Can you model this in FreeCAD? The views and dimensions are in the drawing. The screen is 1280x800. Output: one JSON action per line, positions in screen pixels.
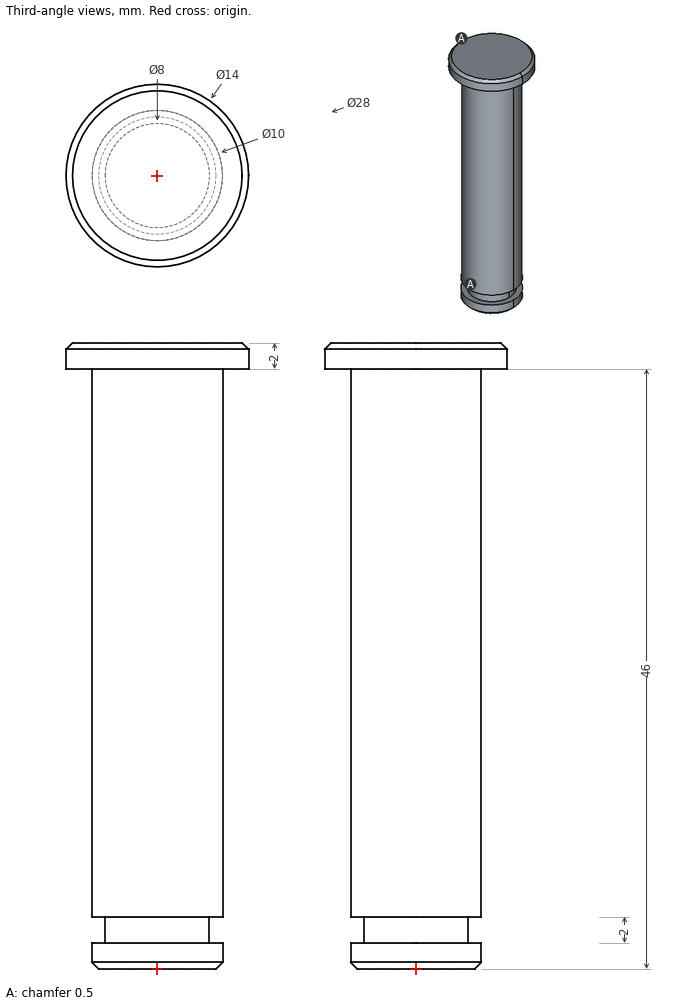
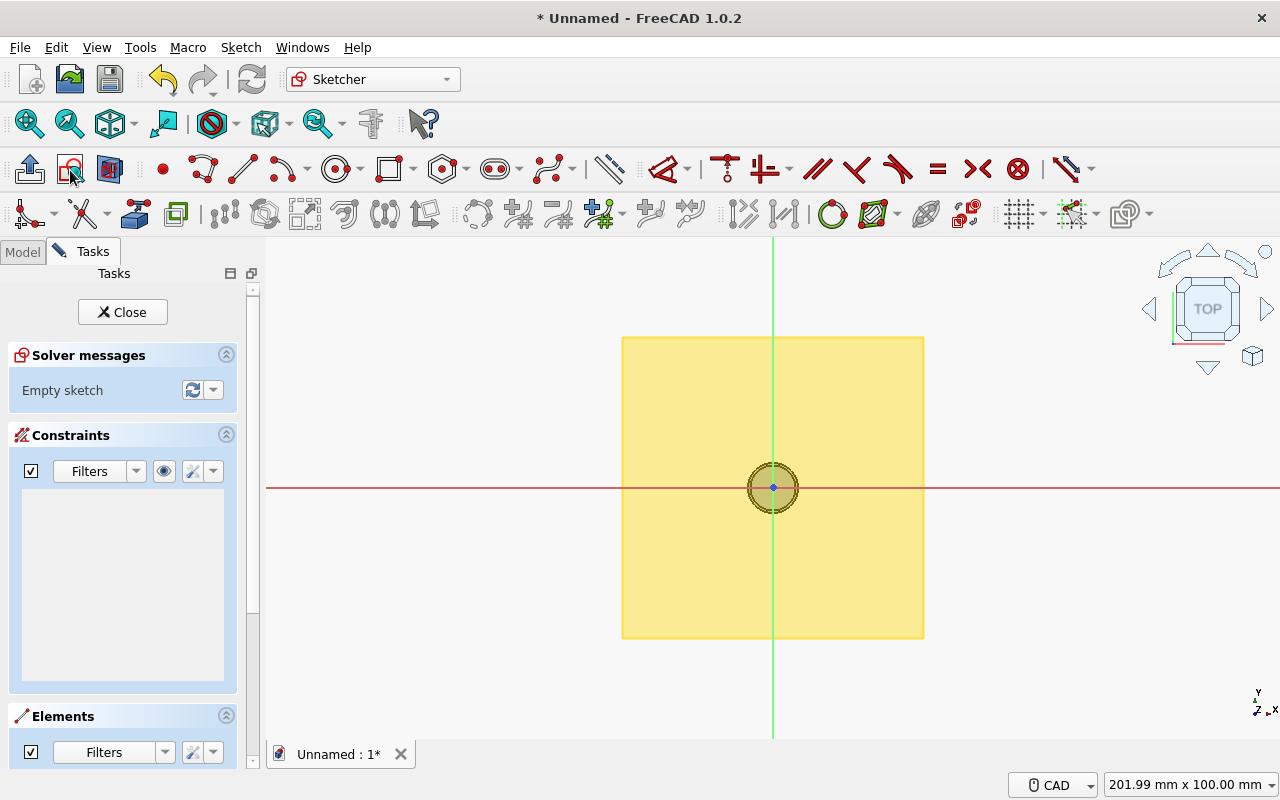
{"action": "scroll", "coordinate": [829, 488], "scroll_direction": "up", "scroll_amount": 4}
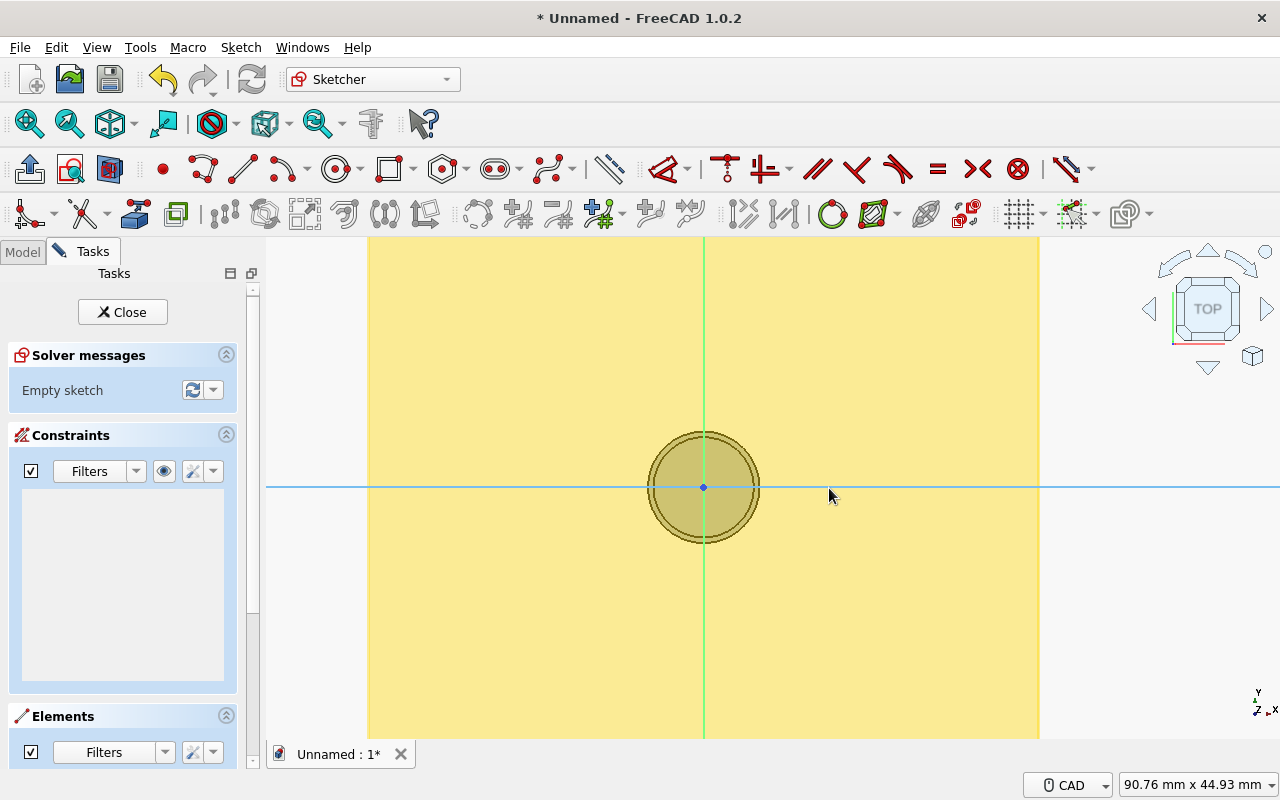
{"action": "left_click", "coordinate": [336, 170]}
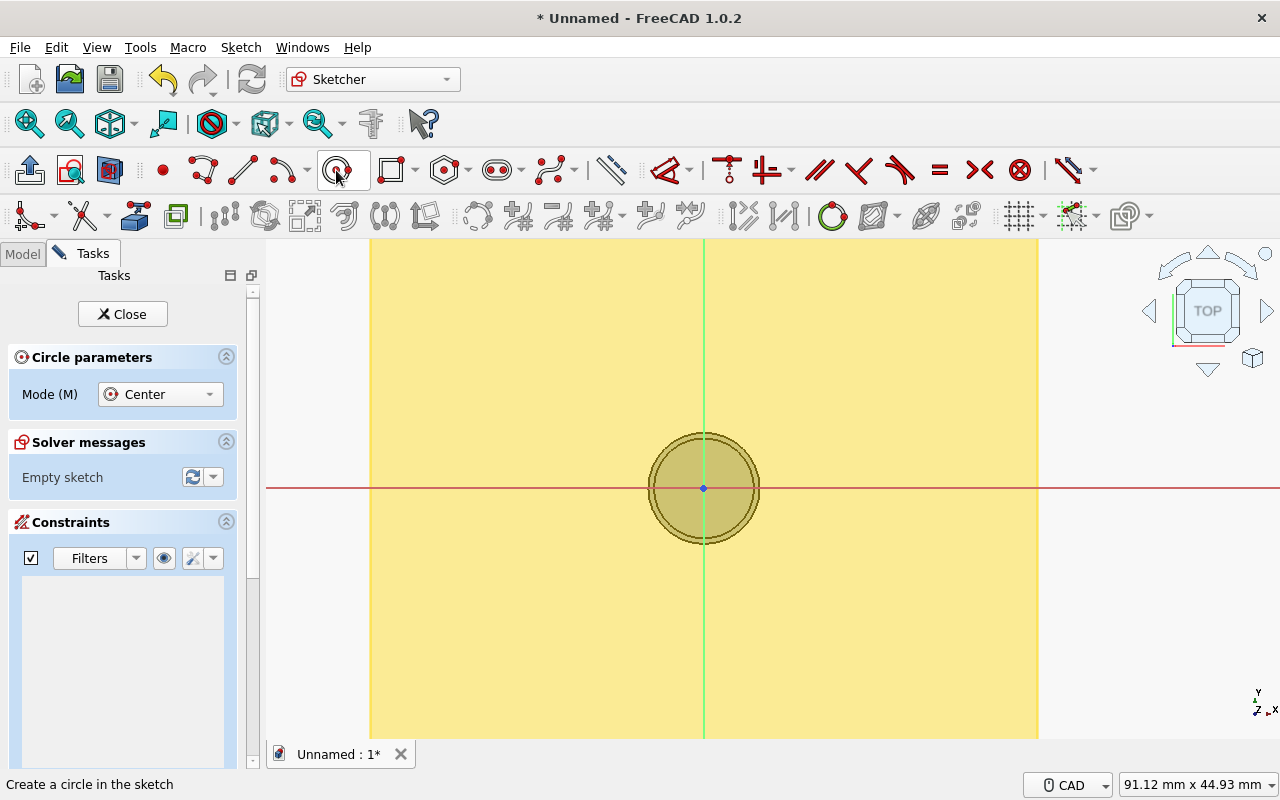
{"action": "left_click", "coordinate": [704, 488]}
{"action": "mouse_move", "coordinate": [814, 378]}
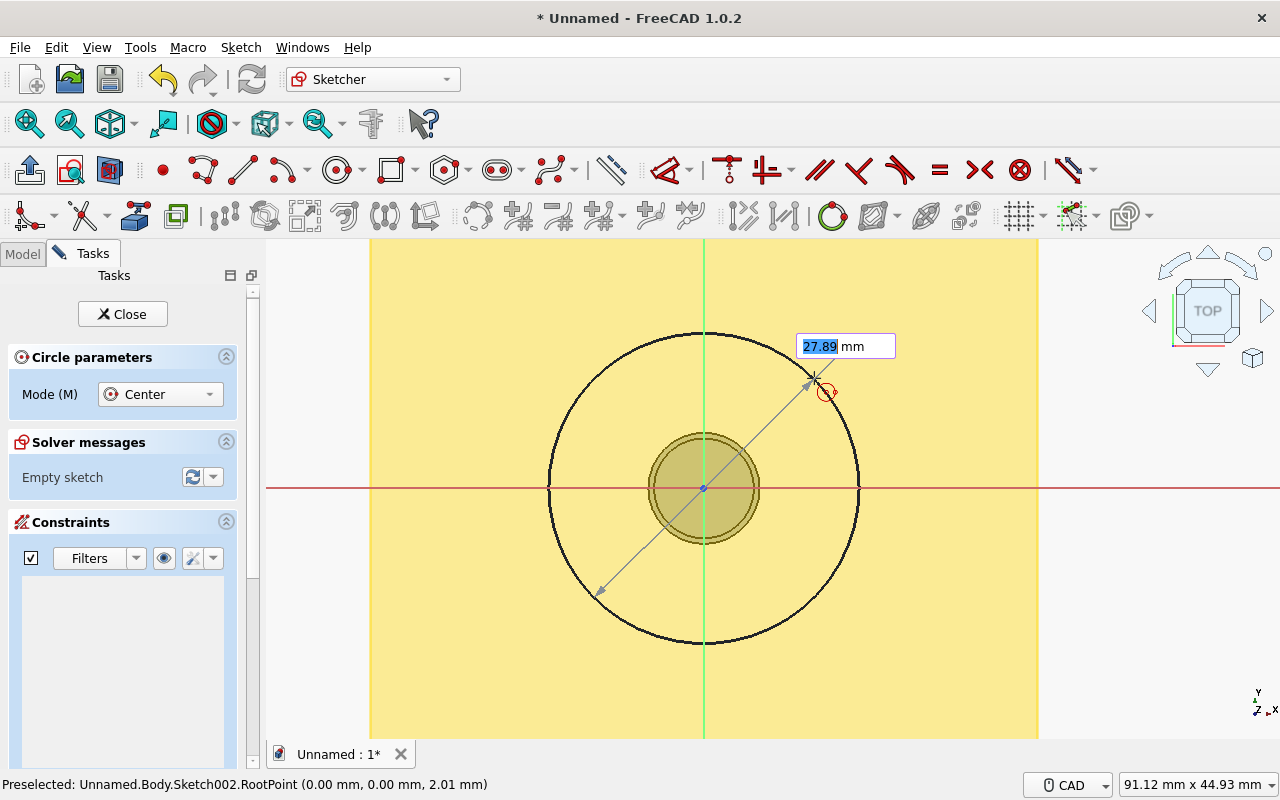
{"action": "type", "text": "28"}
{"action": "key", "text": "Return"}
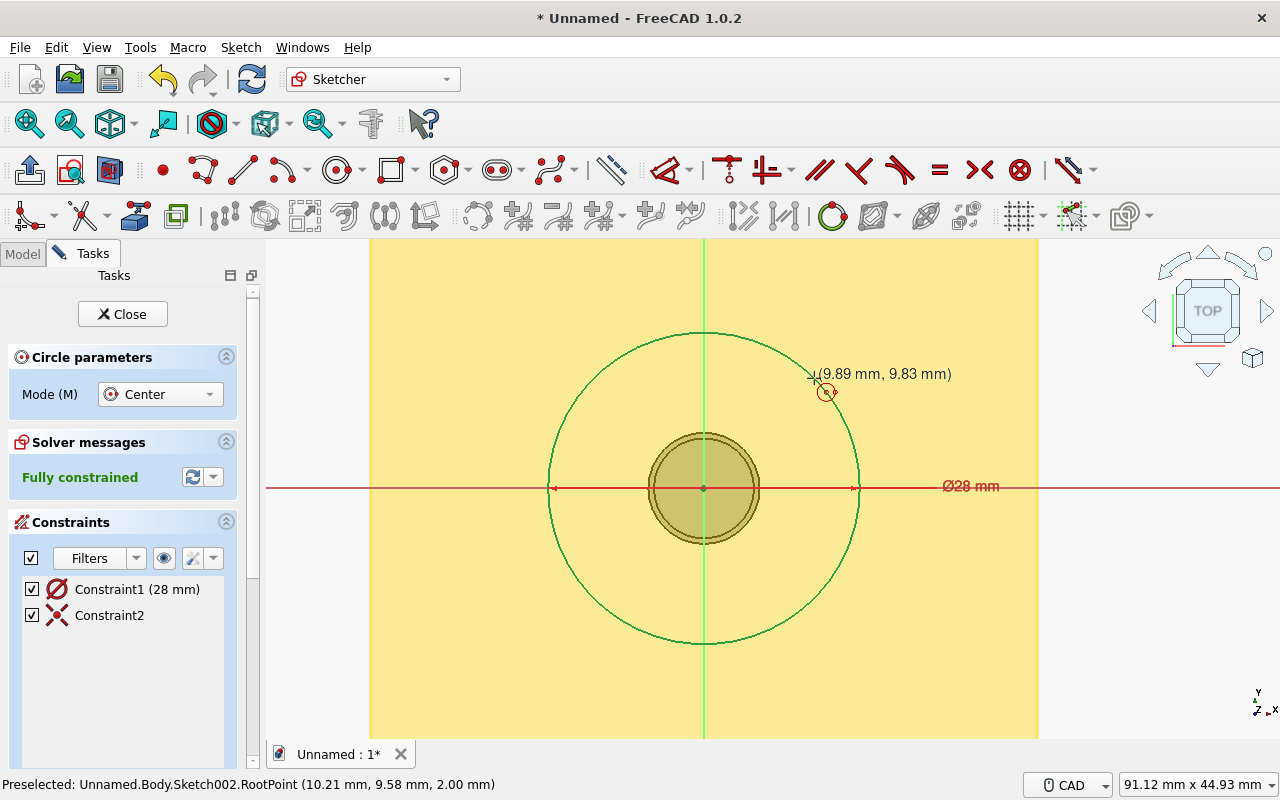
{"action": "left_click", "coordinate": [704, 488]}
{"action": "mouse_move", "coordinate": [735, 457]}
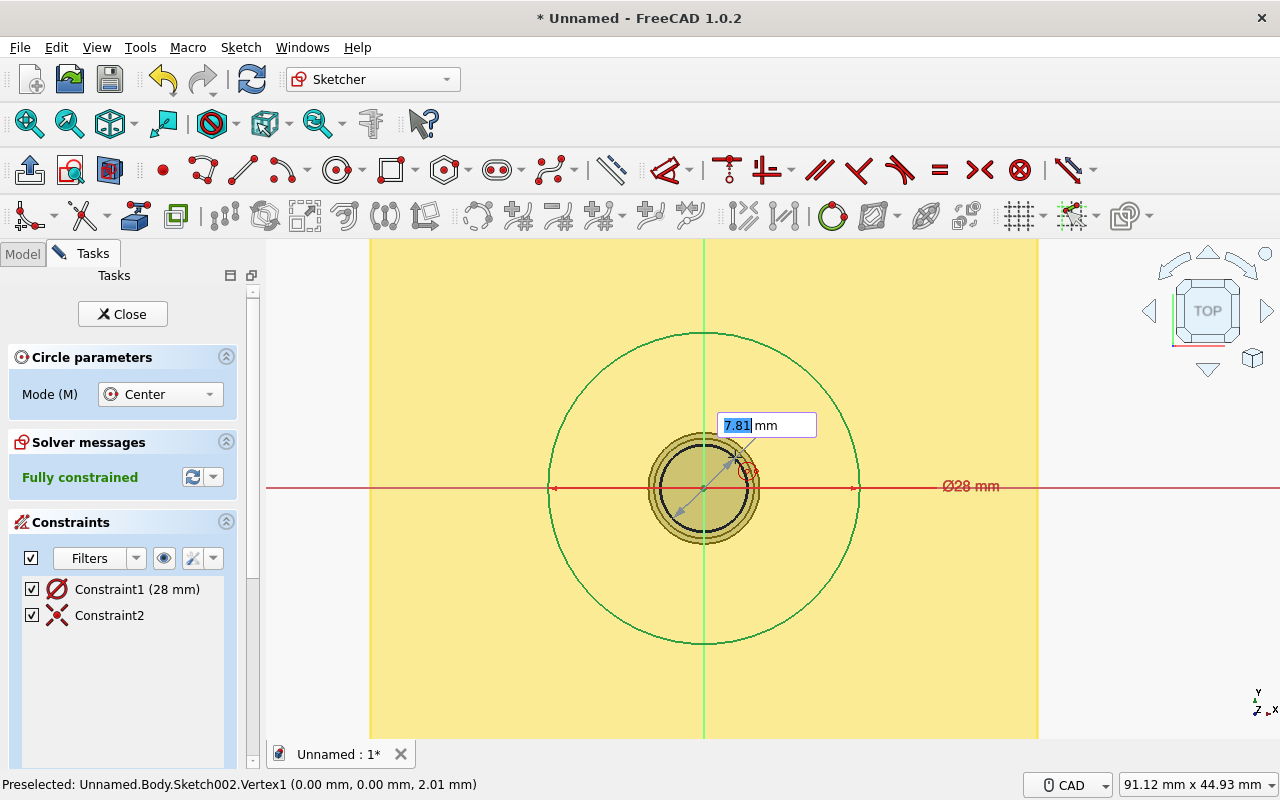
{"action": "type", "text": "8"}
{"action": "key", "text": "Return"}
{"action": "key", "text": "Escape"}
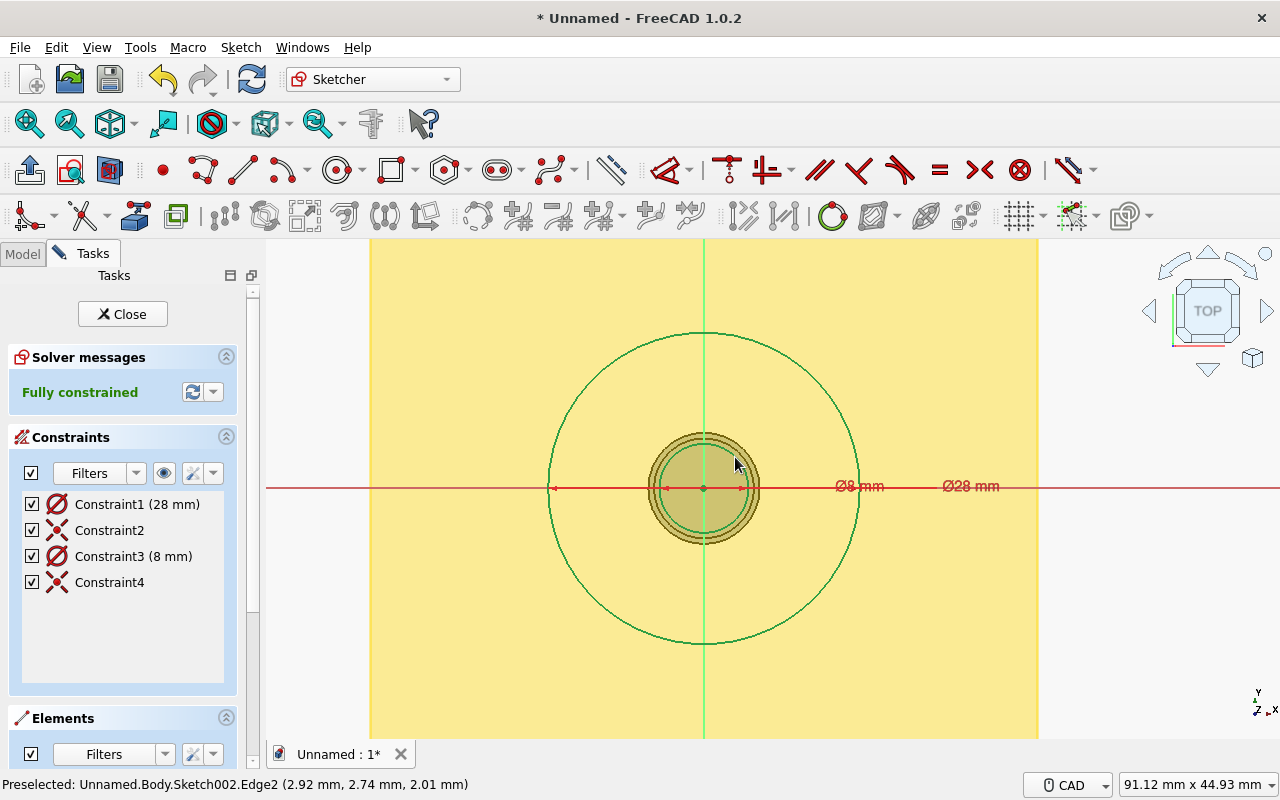
{"action": "left_click", "coordinate": [123, 314]}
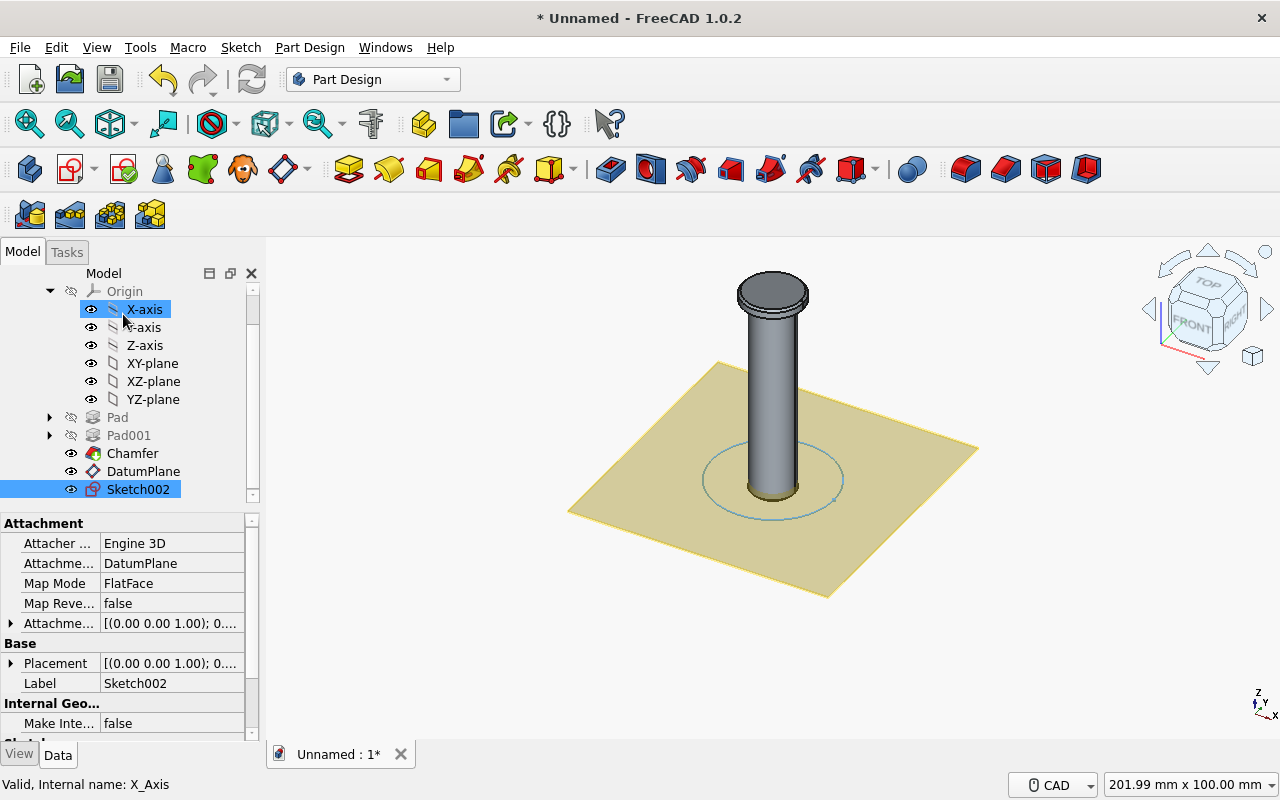
{"action": "left_click", "coordinate": [612, 170]}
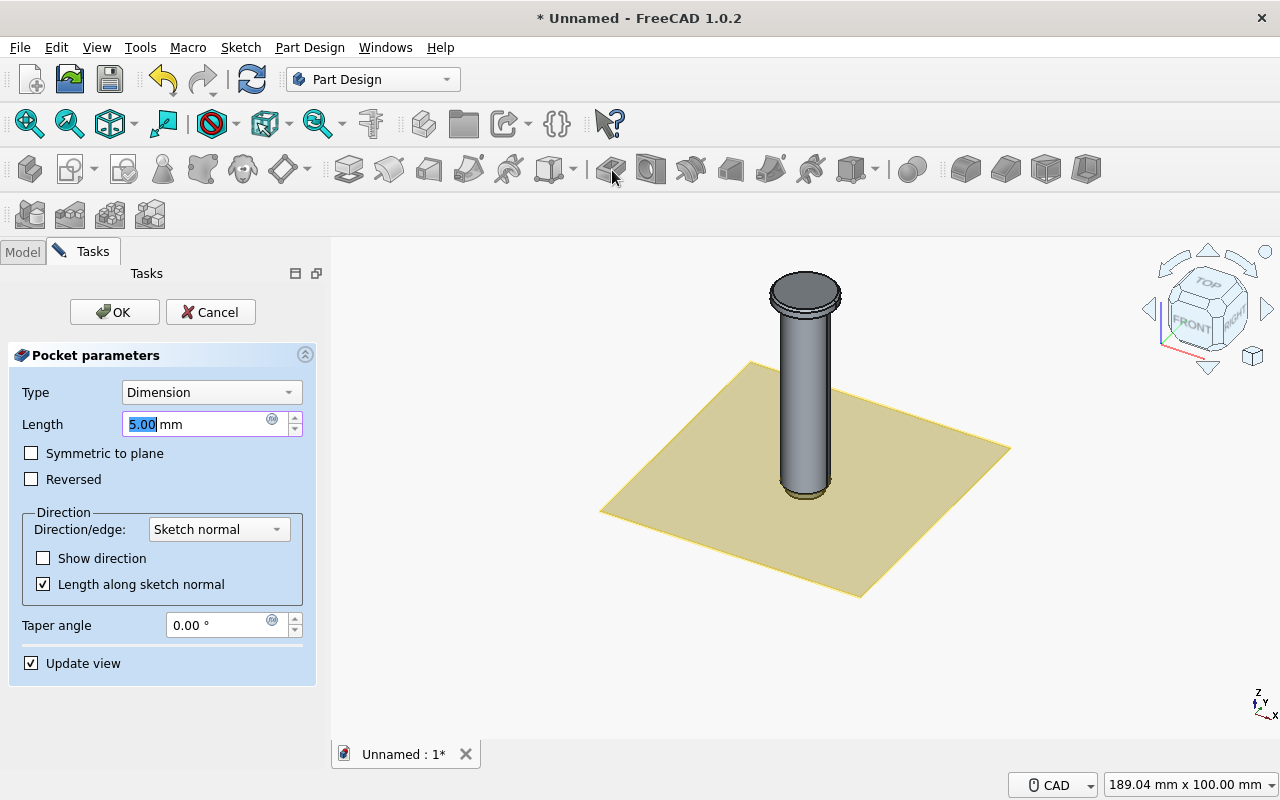
{"action": "type", "text": "2"}
{"action": "key", "text": "Tab"}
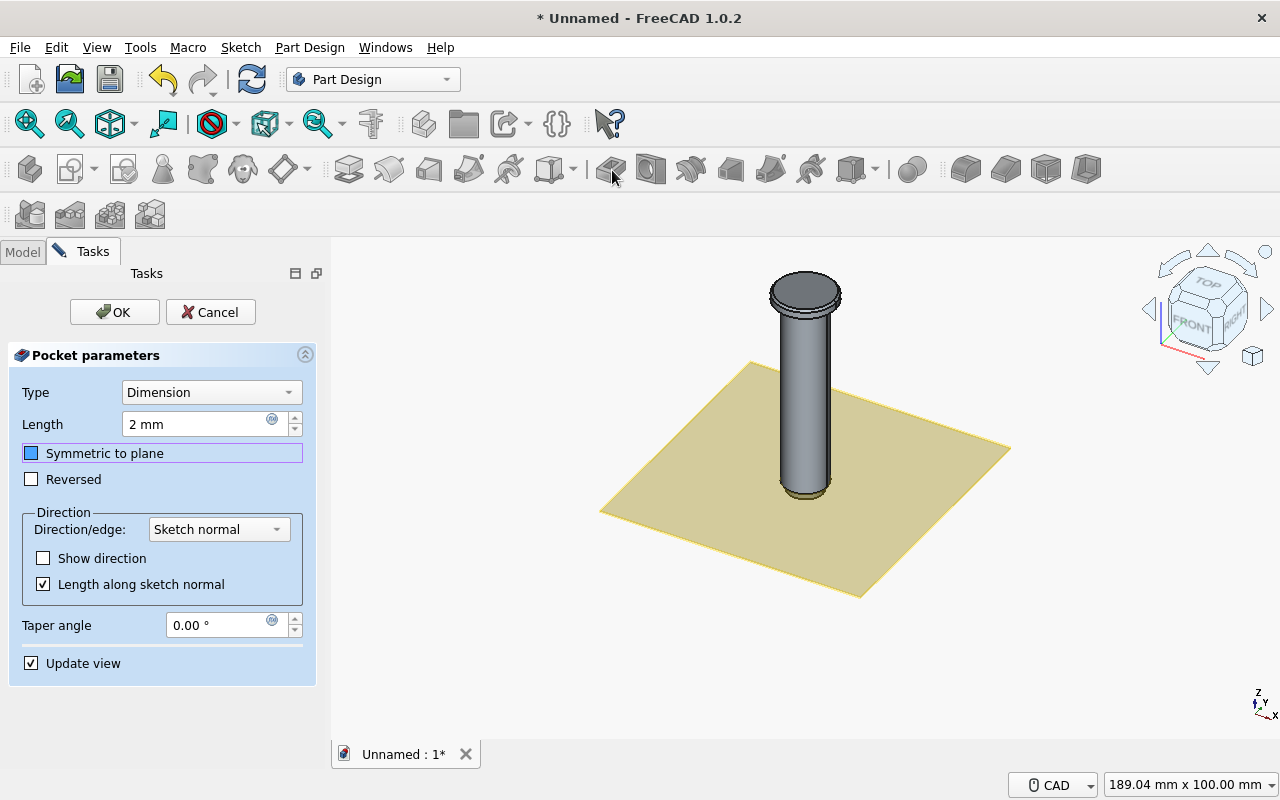
{"action": "left_click", "coordinate": [30, 479]}